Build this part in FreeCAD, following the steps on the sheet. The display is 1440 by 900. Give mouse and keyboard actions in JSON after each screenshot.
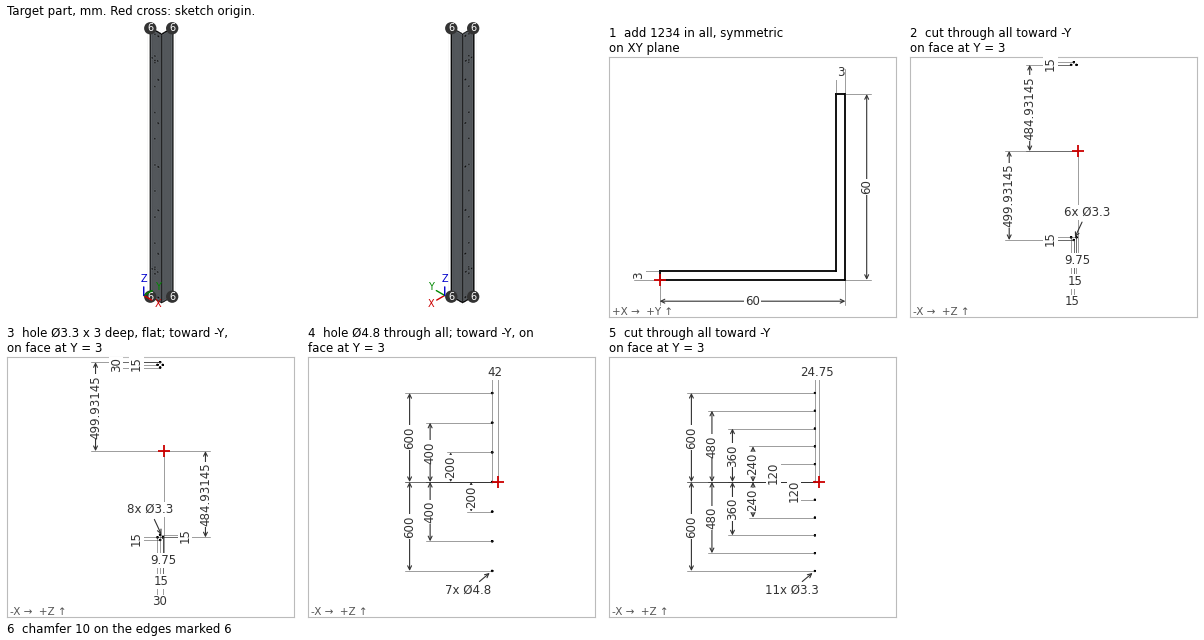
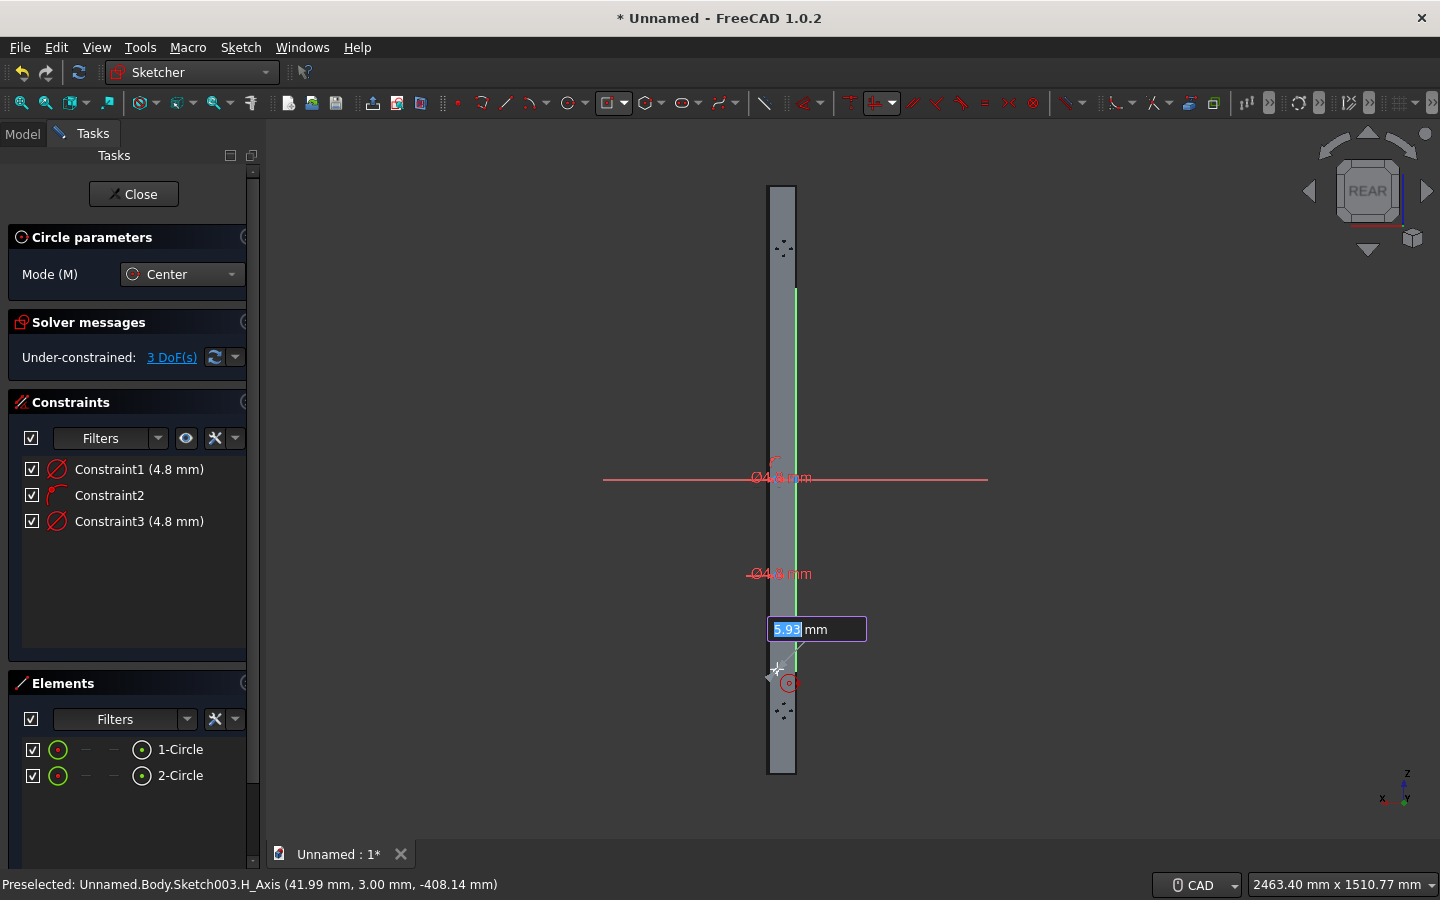
{"action": "type", "text": "4.8"}
{"action": "key", "text": "Return"}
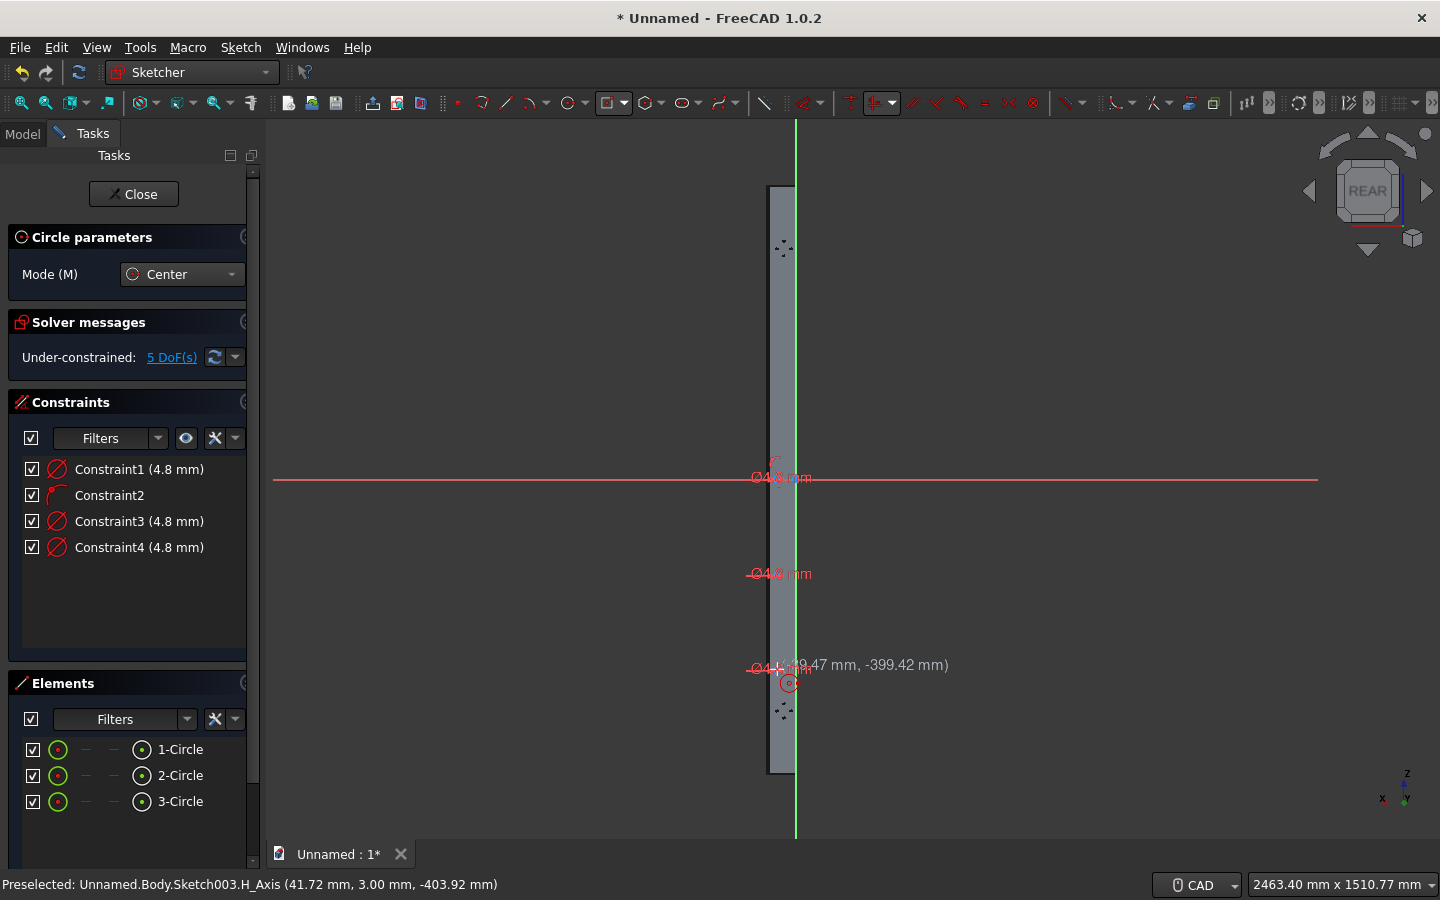
{"action": "scroll", "coordinate": [776, 766], "scroll_direction": "up", "scroll_amount": 15}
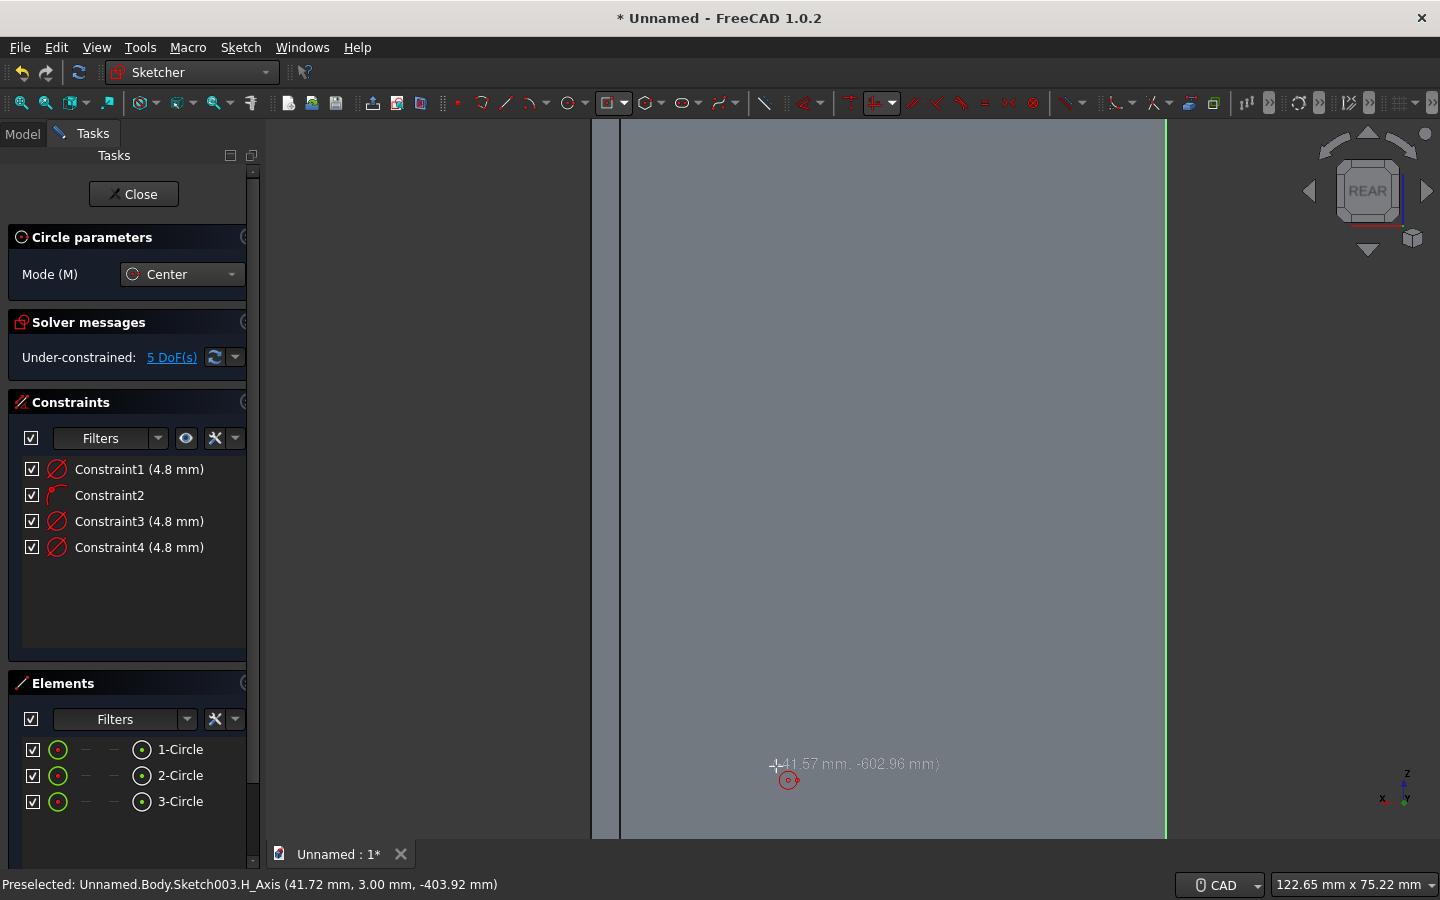
{"action": "scroll", "coordinate": [776, 766], "scroll_direction": "down", "scroll_amount": 15}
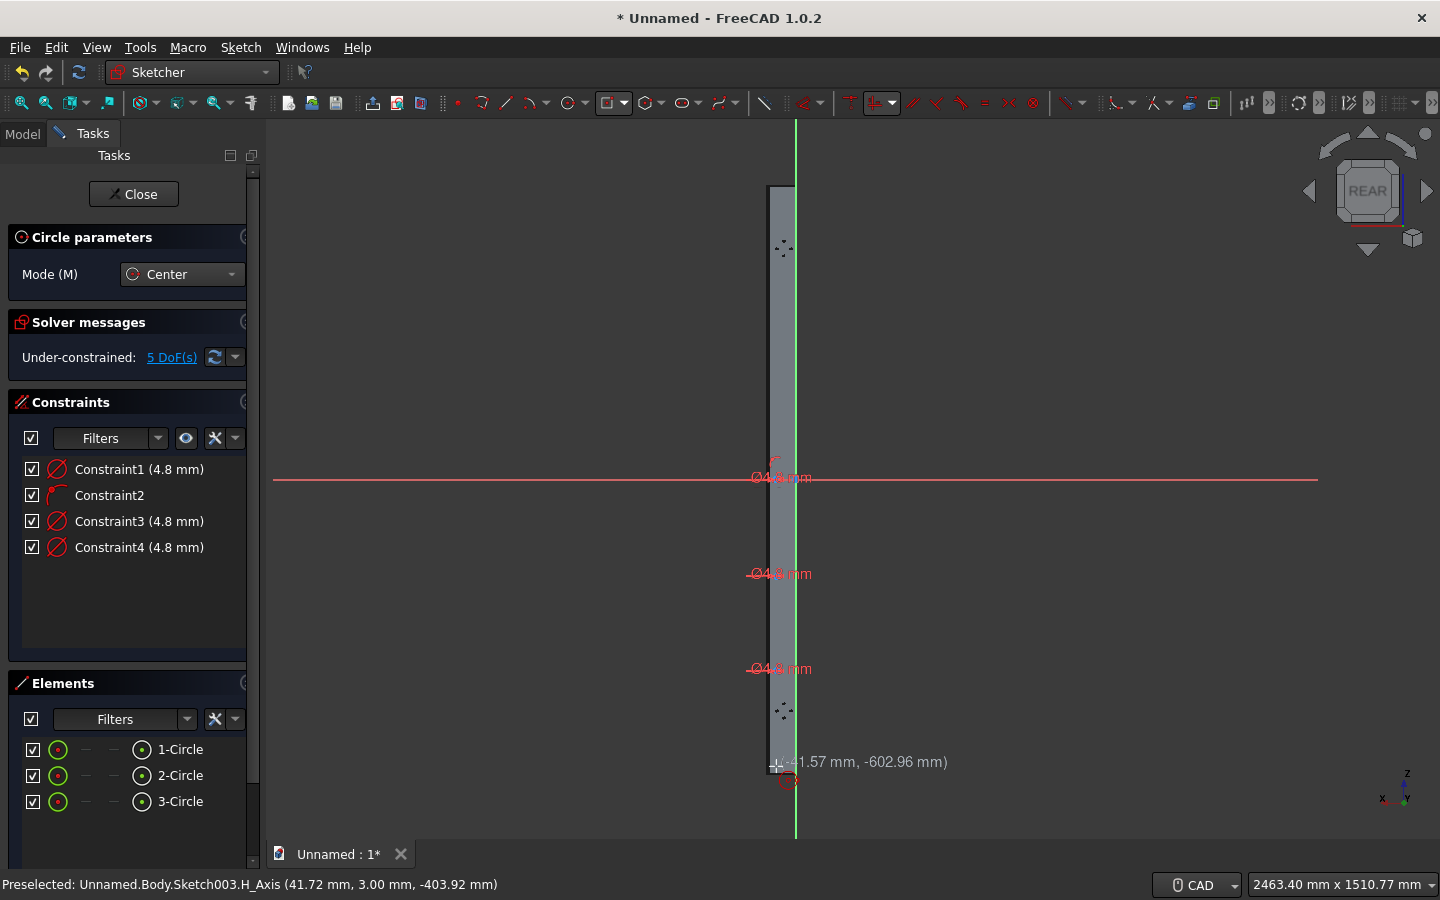
{"action": "left_click", "coordinate": [776, 766]}
{"action": "mouse_move", "coordinate": [777, 765]}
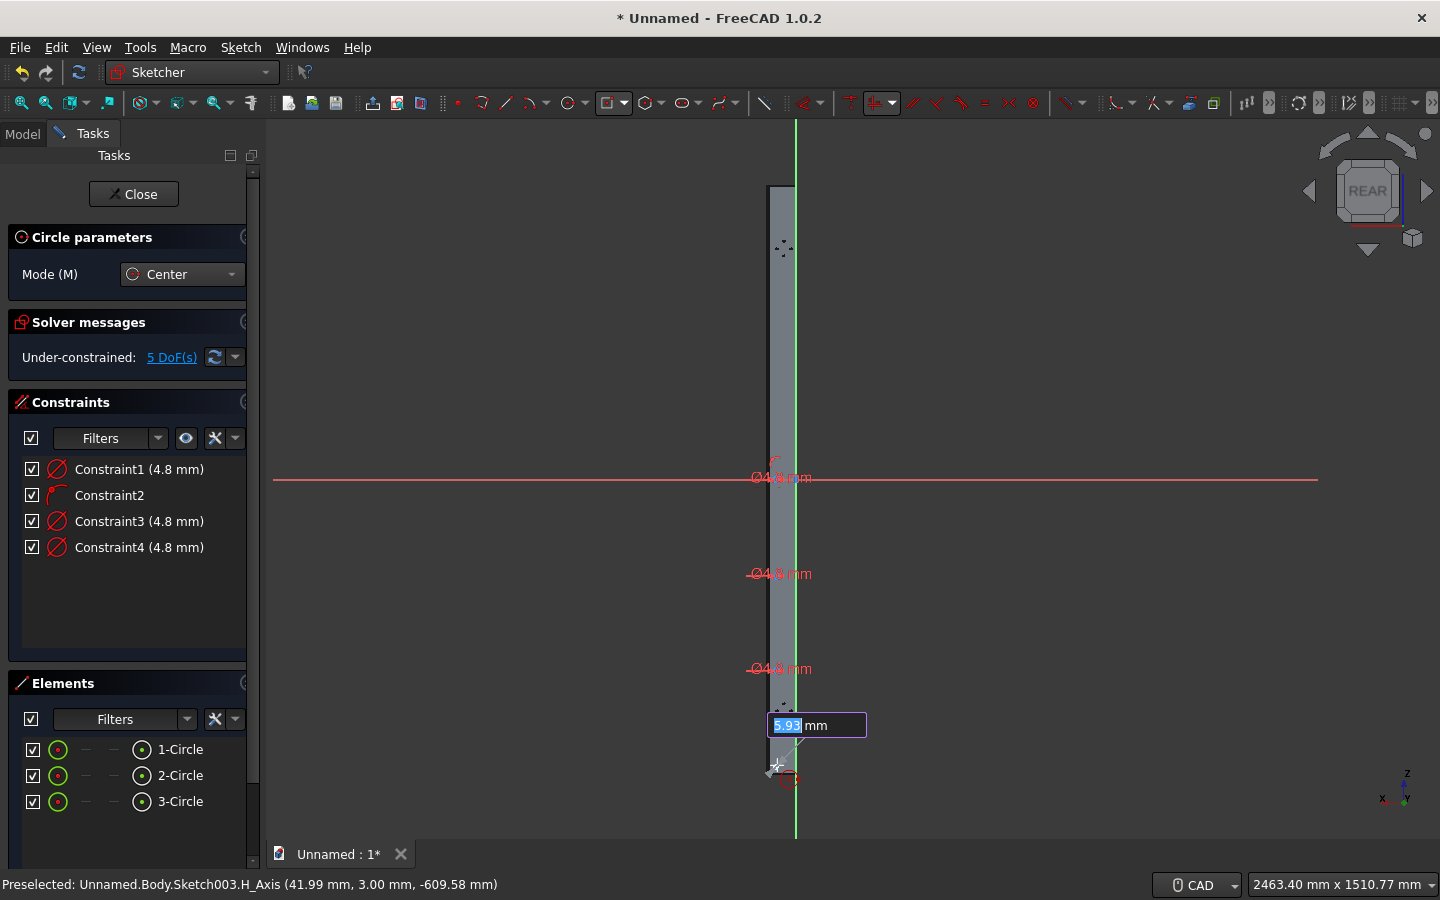
{"action": "type", "text": "4.8"}
{"action": "key", "text": "Return"}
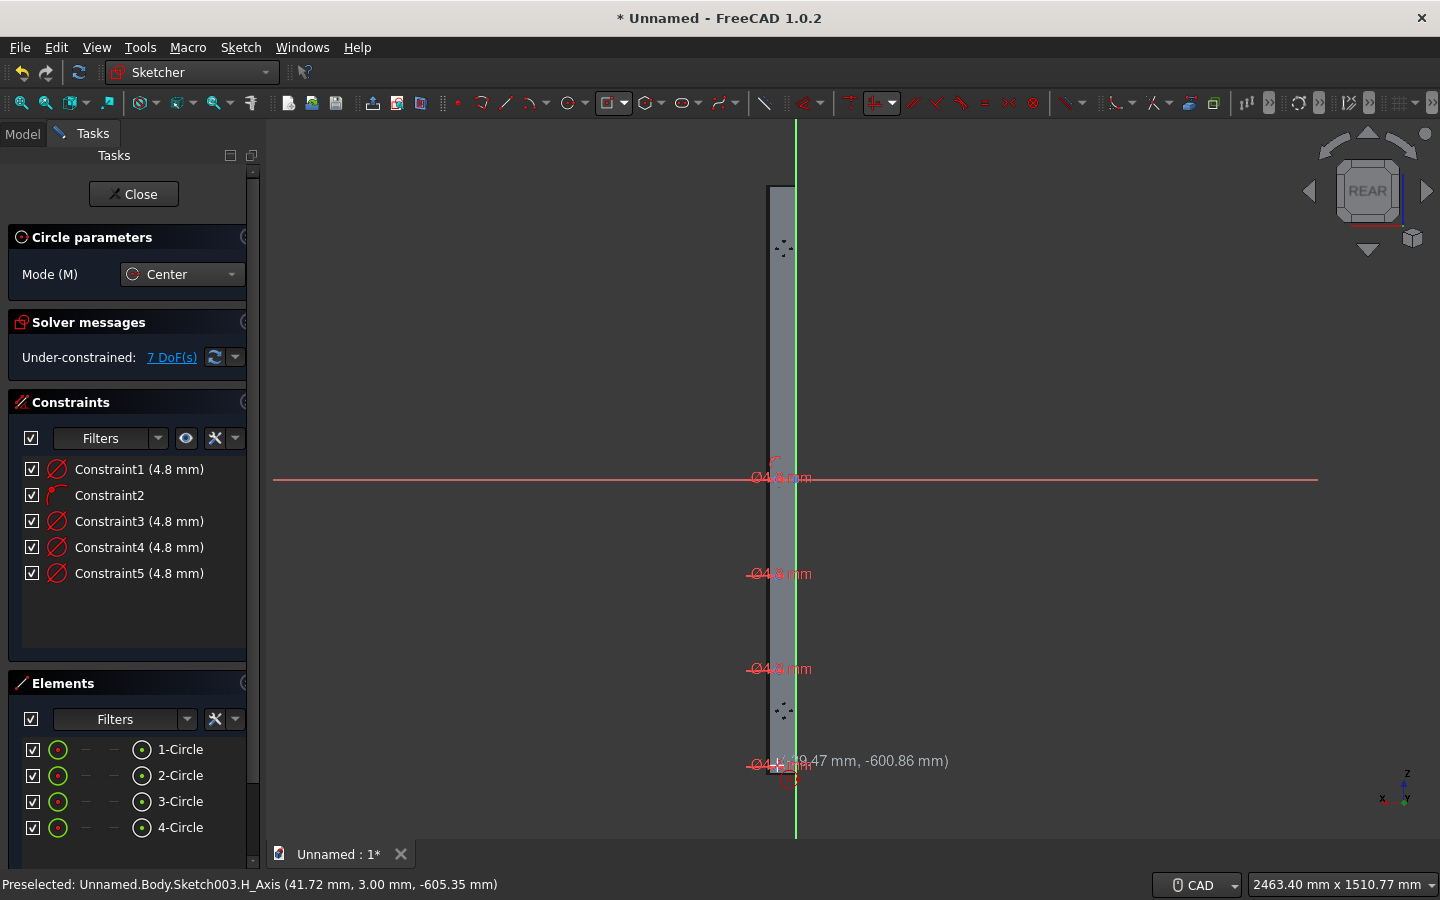
{"action": "scroll", "coordinate": [776, 194], "scroll_direction": "up", "scroll_amount": 15}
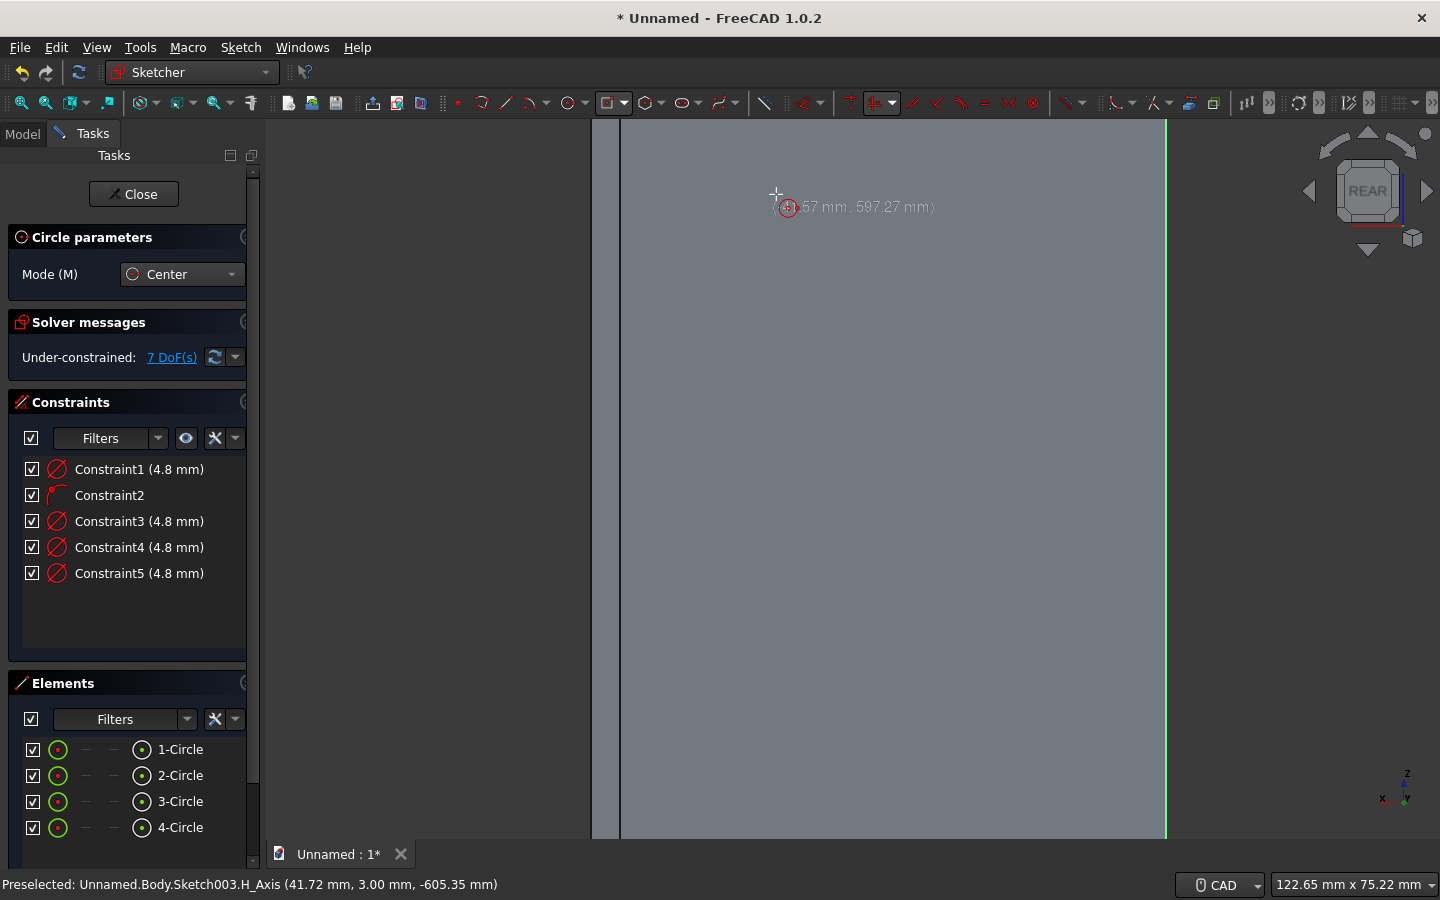
{"action": "scroll", "coordinate": [776, 193], "scroll_direction": "down", "scroll_amount": 15}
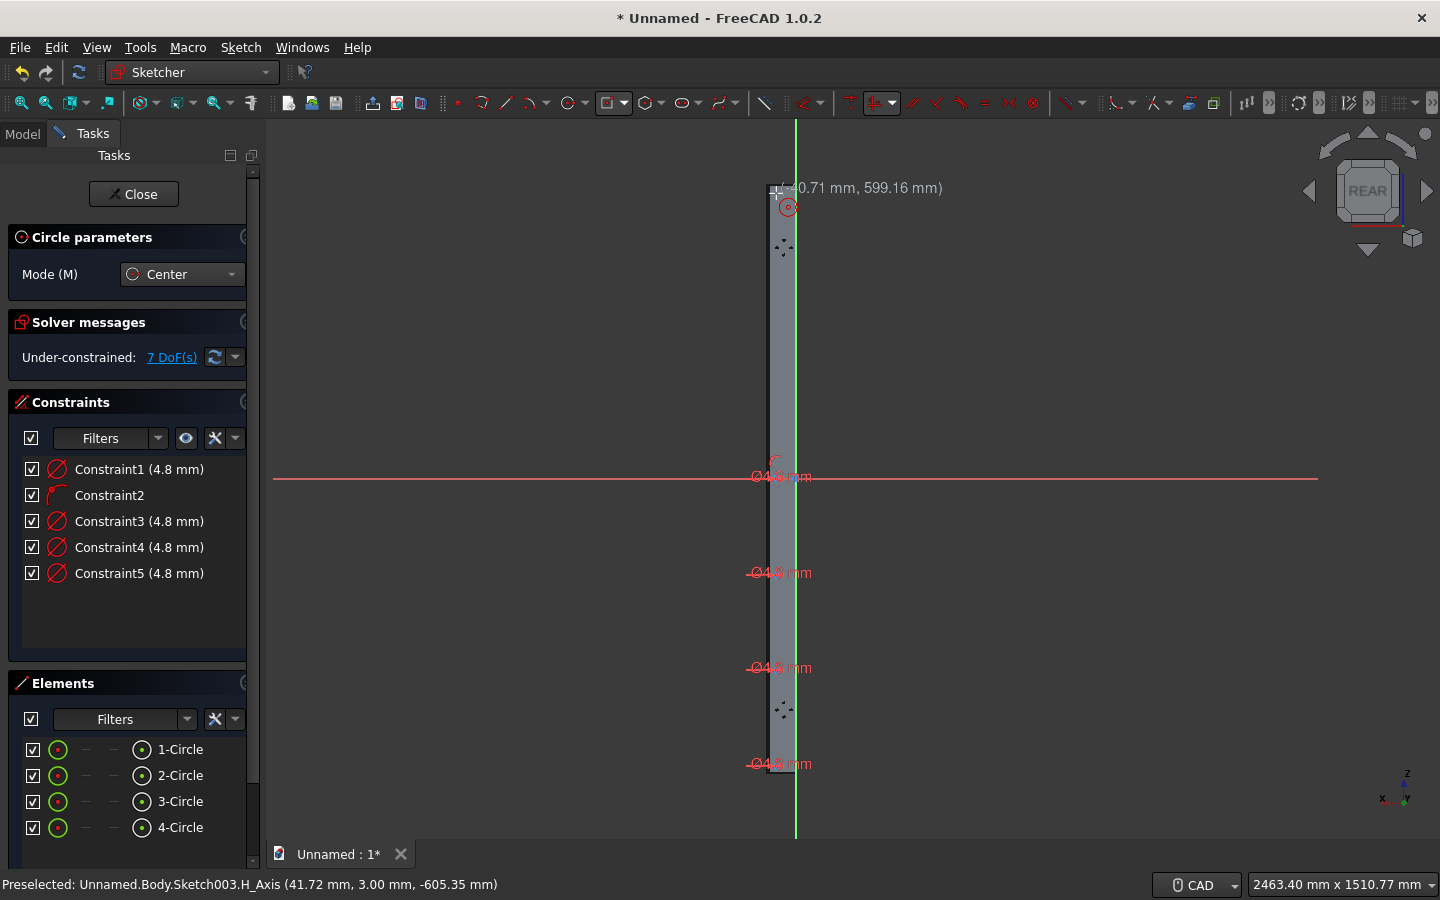
{"action": "left_click", "coordinate": [776, 193]}
{"action": "mouse_move", "coordinate": [777, 192]}